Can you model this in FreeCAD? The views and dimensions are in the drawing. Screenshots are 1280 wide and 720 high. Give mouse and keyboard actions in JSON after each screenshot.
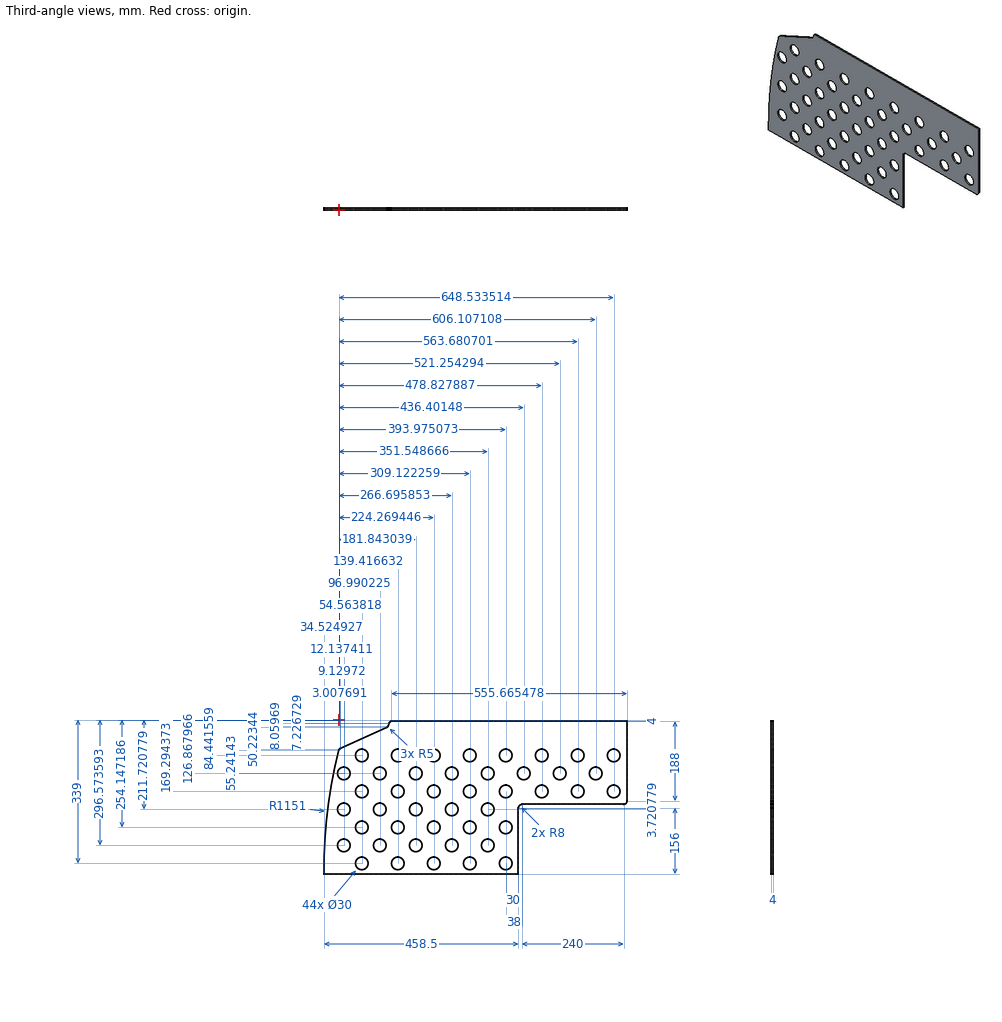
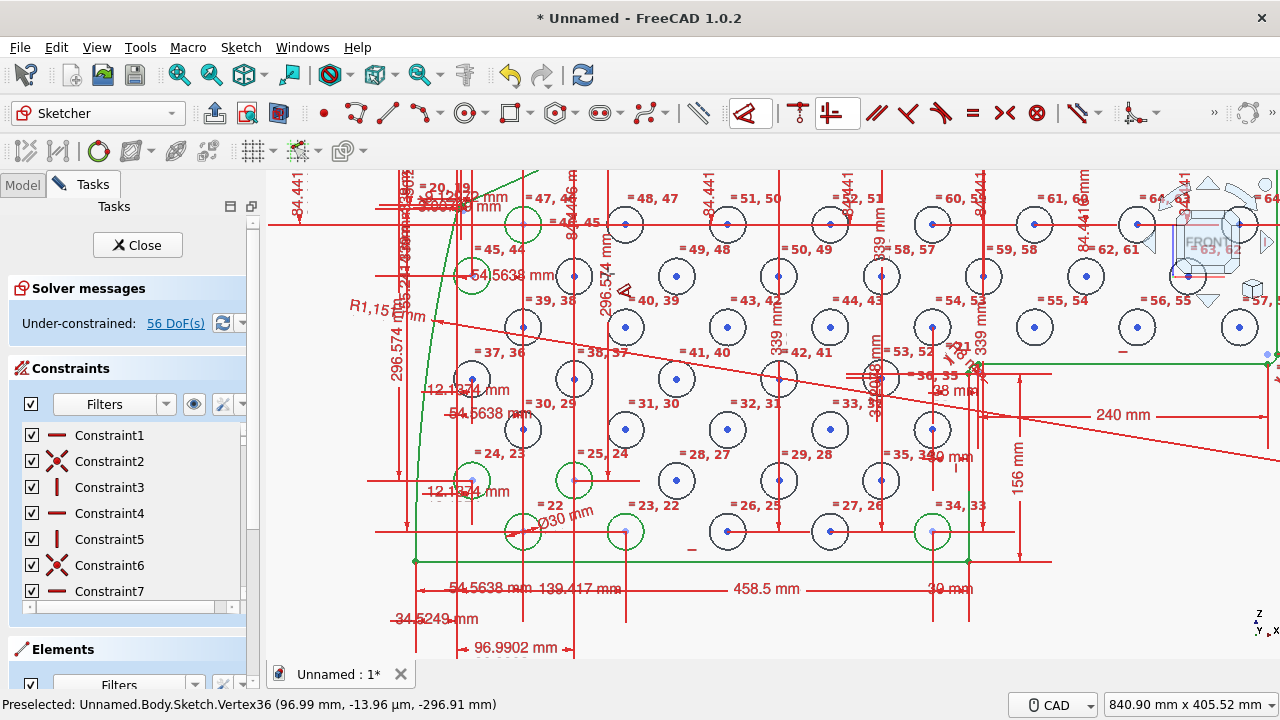
{"action": "left_click", "coordinate": [728, 532]}
{"action": "left_click", "coordinate": [655, 590]}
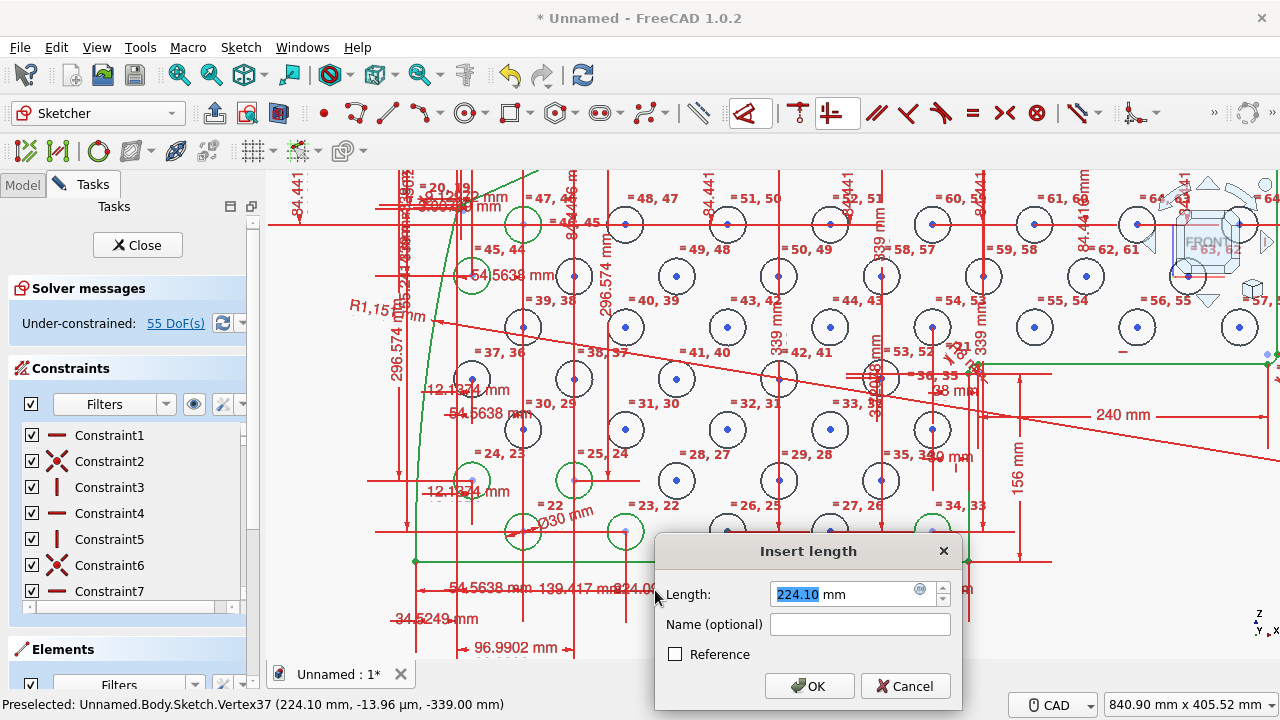
{"action": "type", "text": "224.269446"}
{"action": "key", "text": "Return"}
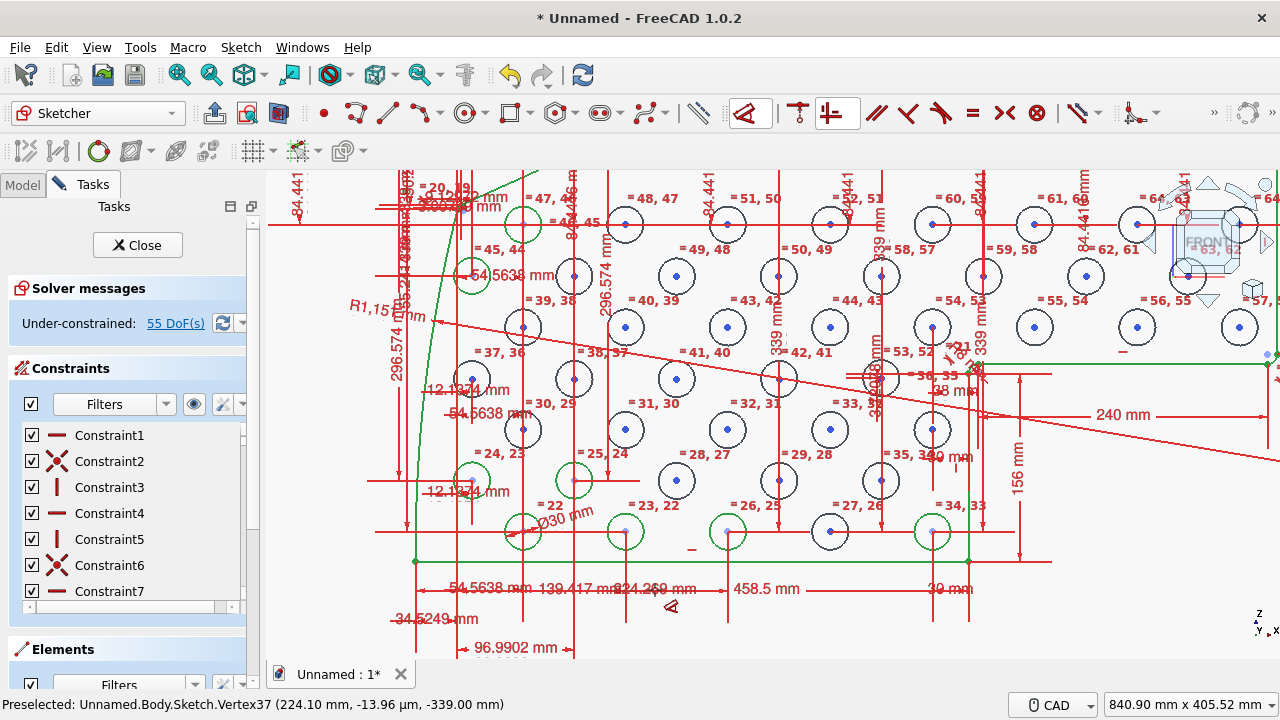
{"action": "left_click", "coordinate": [830, 532]}
{"action": "left_click", "coordinate": [644, 614]}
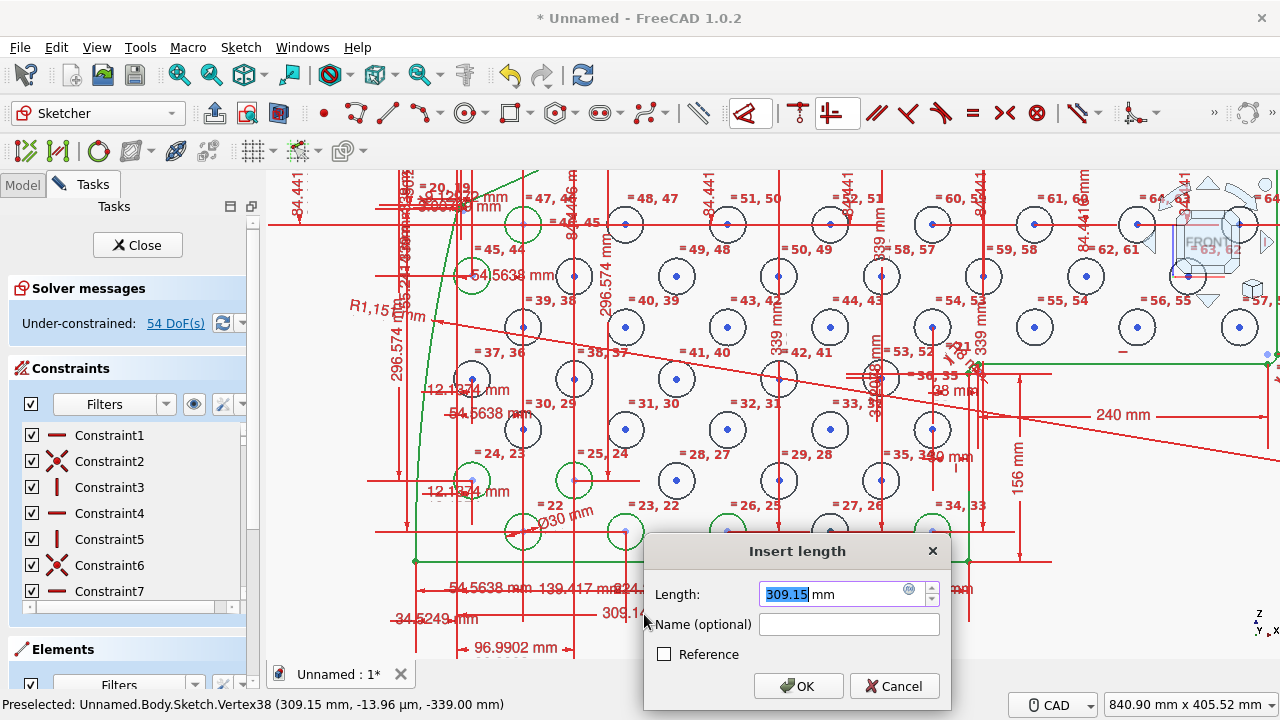
{"action": "type", "text": "309.122259"}
{"action": "key", "text": "Return"}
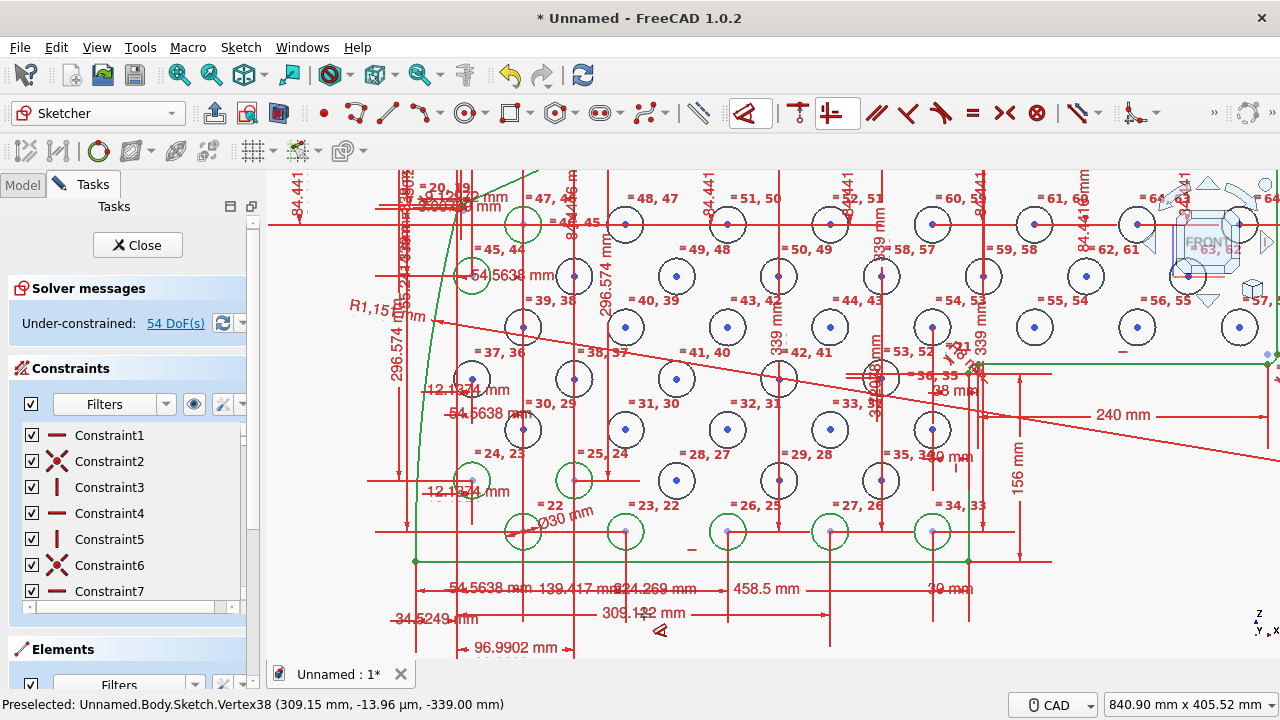
{"action": "left_click", "coordinate": [677, 481]}
{"action": "left_click", "coordinate": [490, 515]}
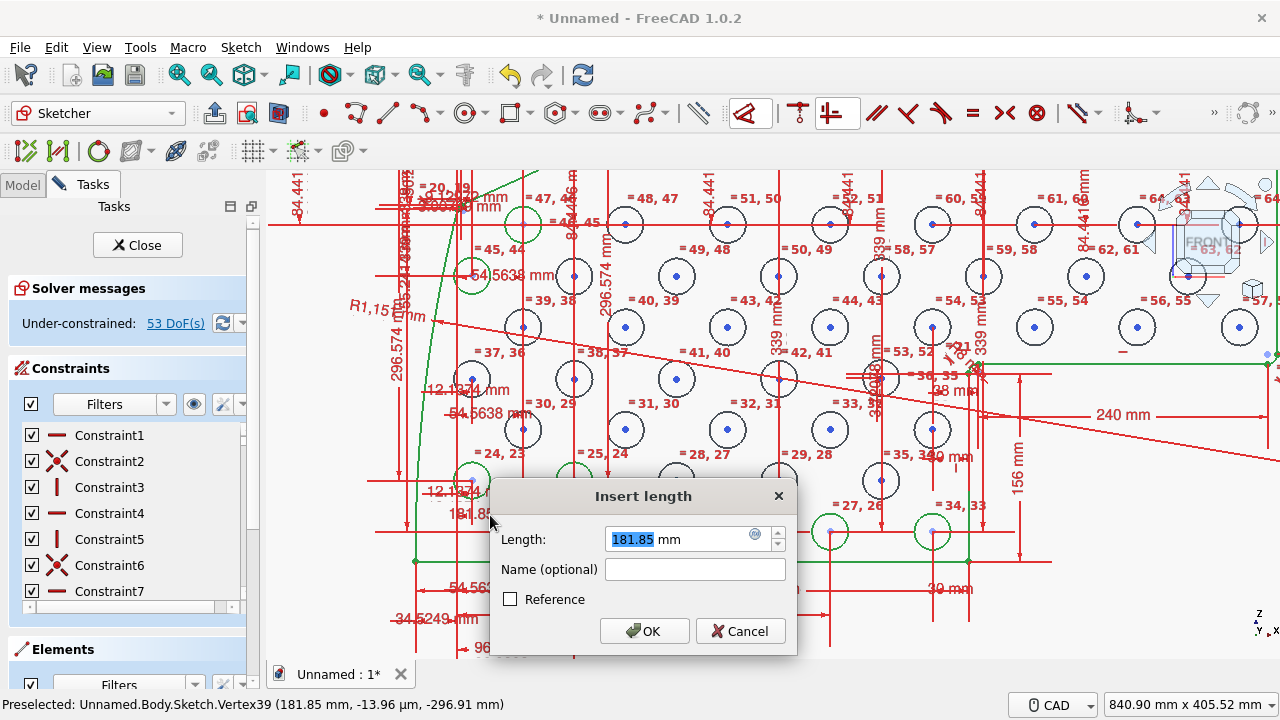
{"action": "type", "text": "181.843039"}
{"action": "key", "text": "Return"}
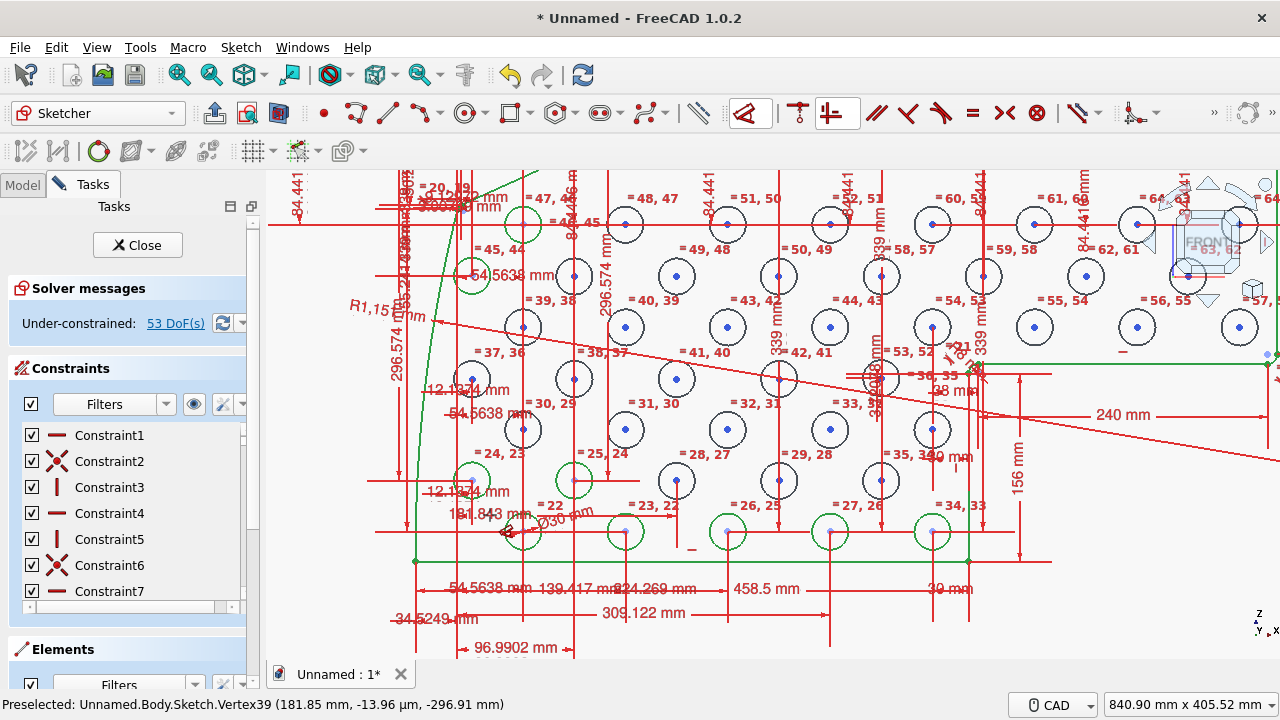
{"action": "left_click", "coordinate": [677, 481]}
{"action": "left_click", "coordinate": [711, 274]}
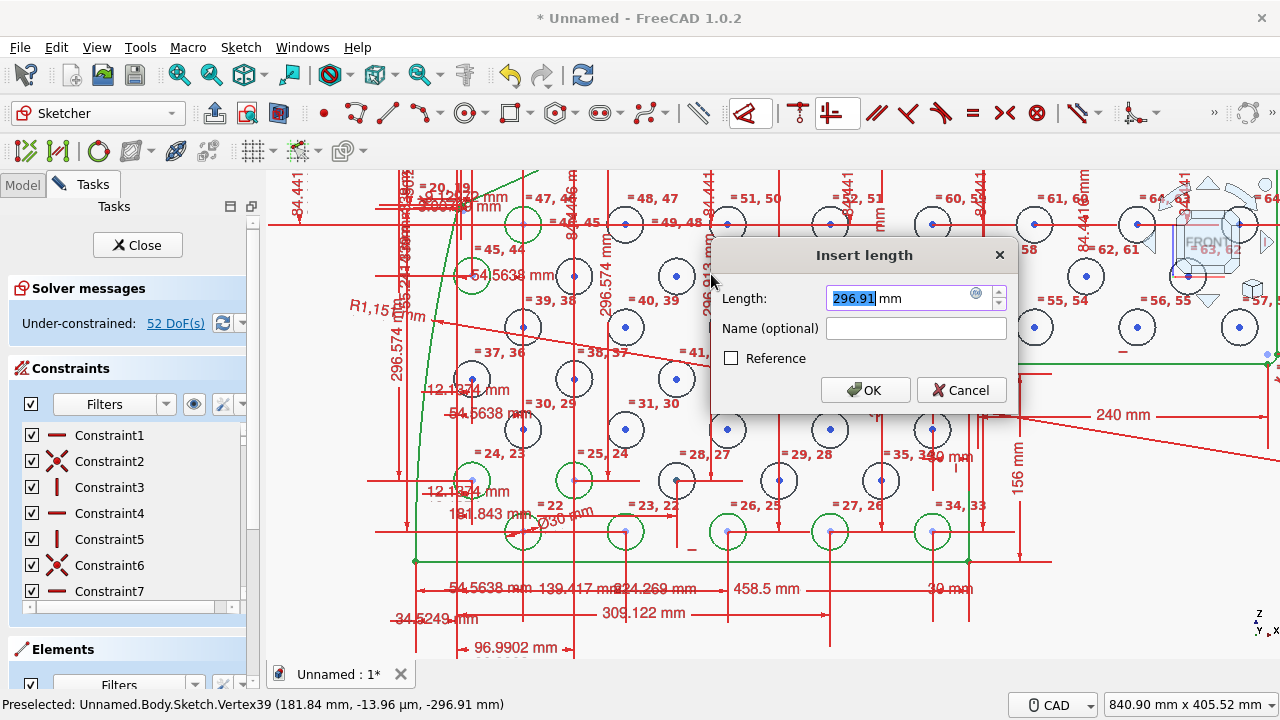
{"action": "type", "text": "296.573593"}
{"action": "key", "text": "Return"}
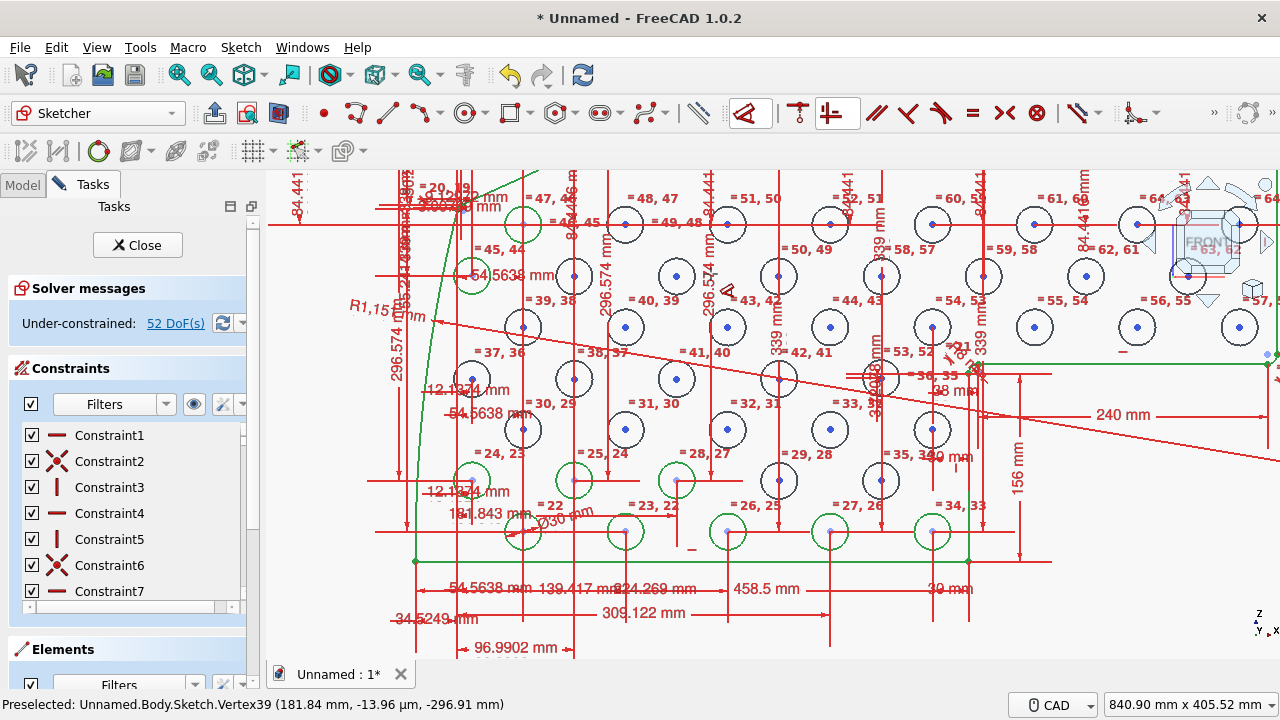
{"action": "left_click", "coordinate": [779, 481]}
{"action": "left_click", "coordinate": [692, 515]}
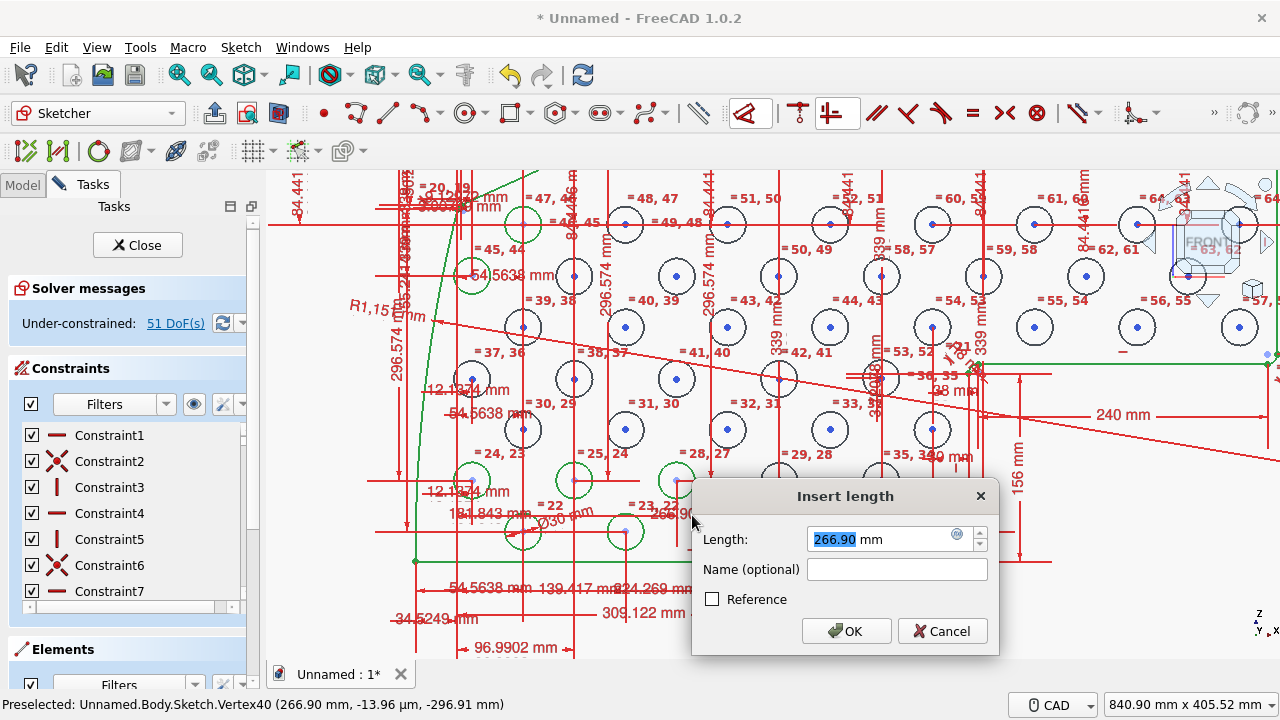
{"action": "type", "text": "266.695853"}
{"action": "key", "text": "Return"}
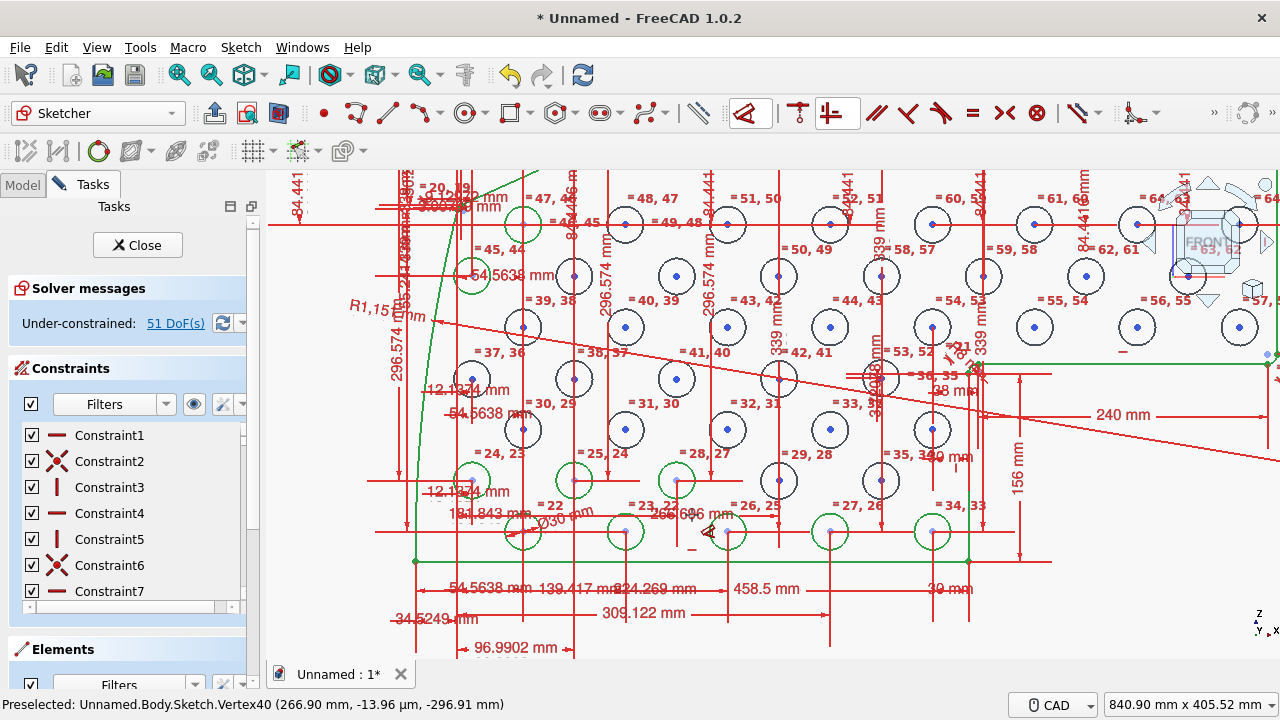
{"action": "left_click", "coordinate": [779, 481]}
{"action": "left_click", "coordinate": [813, 274]}